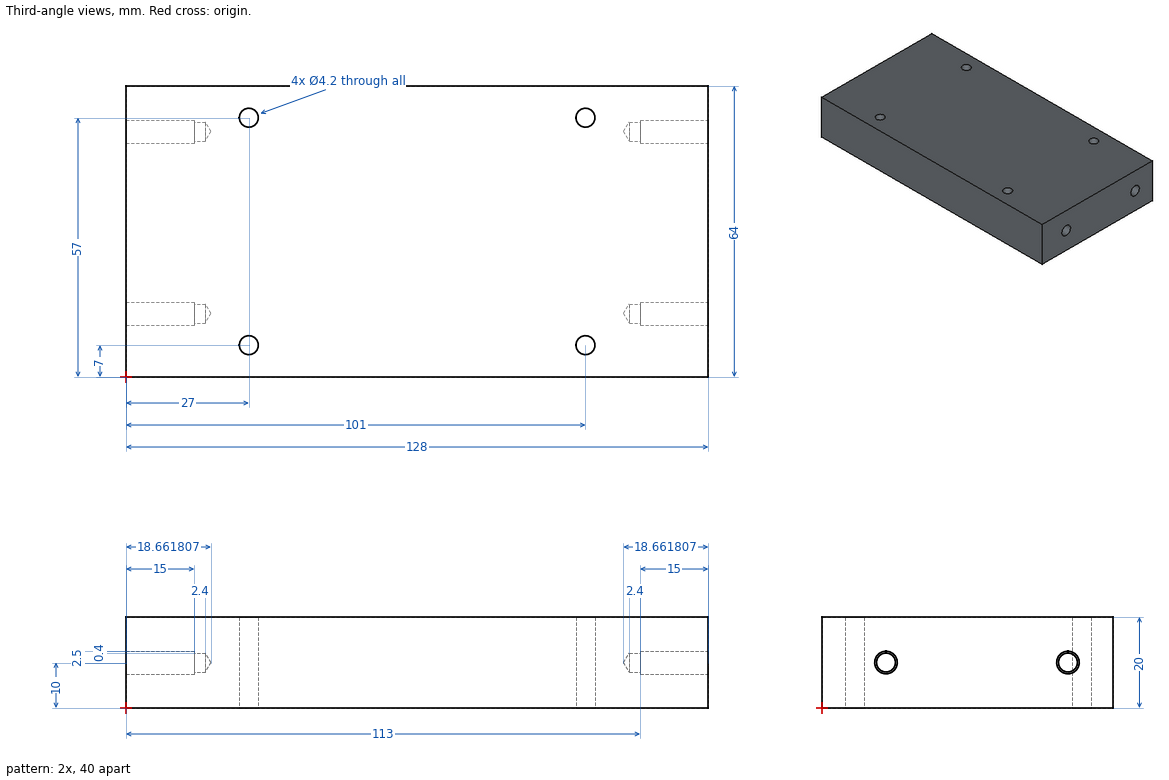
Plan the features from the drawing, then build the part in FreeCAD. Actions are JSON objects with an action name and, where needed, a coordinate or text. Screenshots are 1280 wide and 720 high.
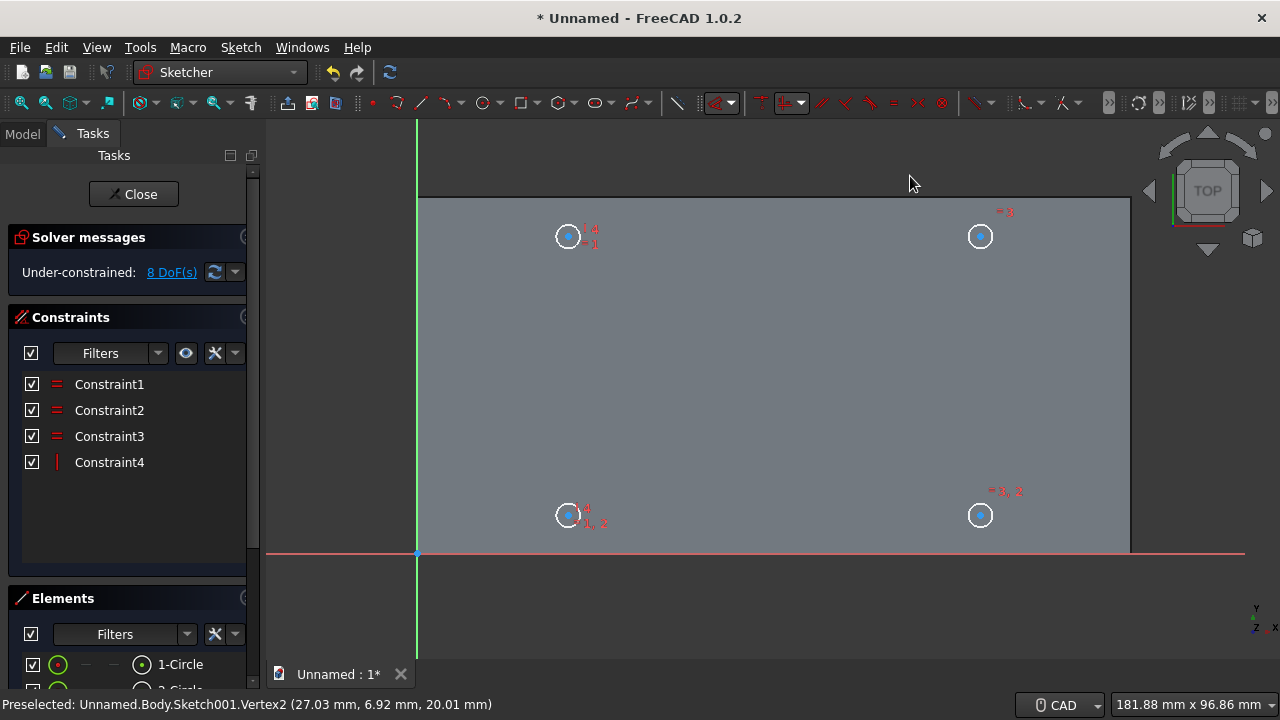
{"action": "left_click", "coordinate": [568, 515]}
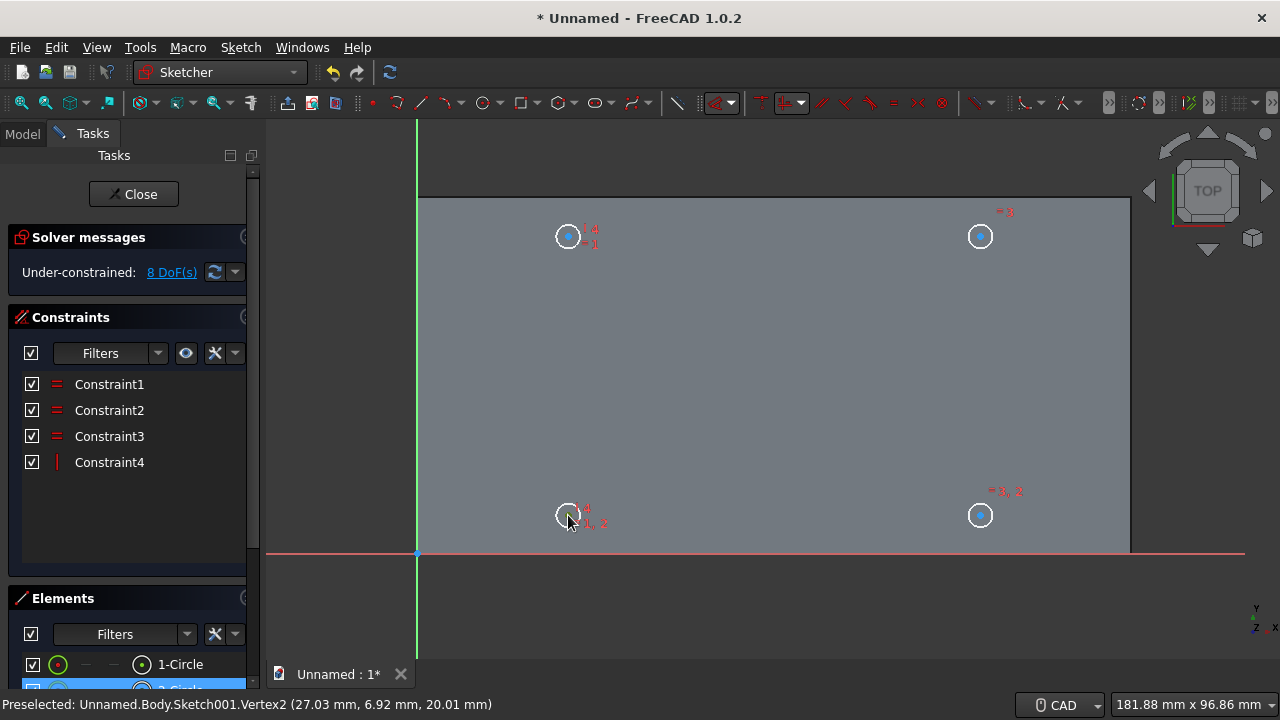
{"action": "left_click", "coordinate": [980, 515]}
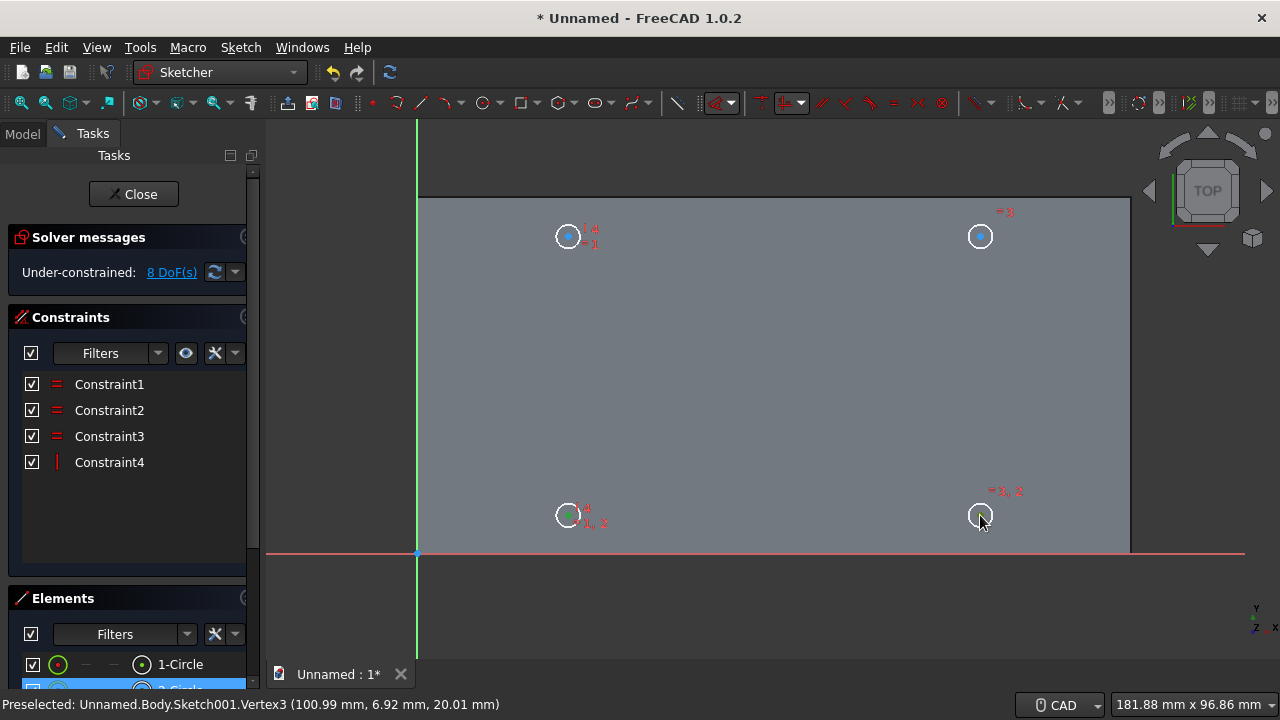
{"action": "left_click", "coordinate": [804, 104]}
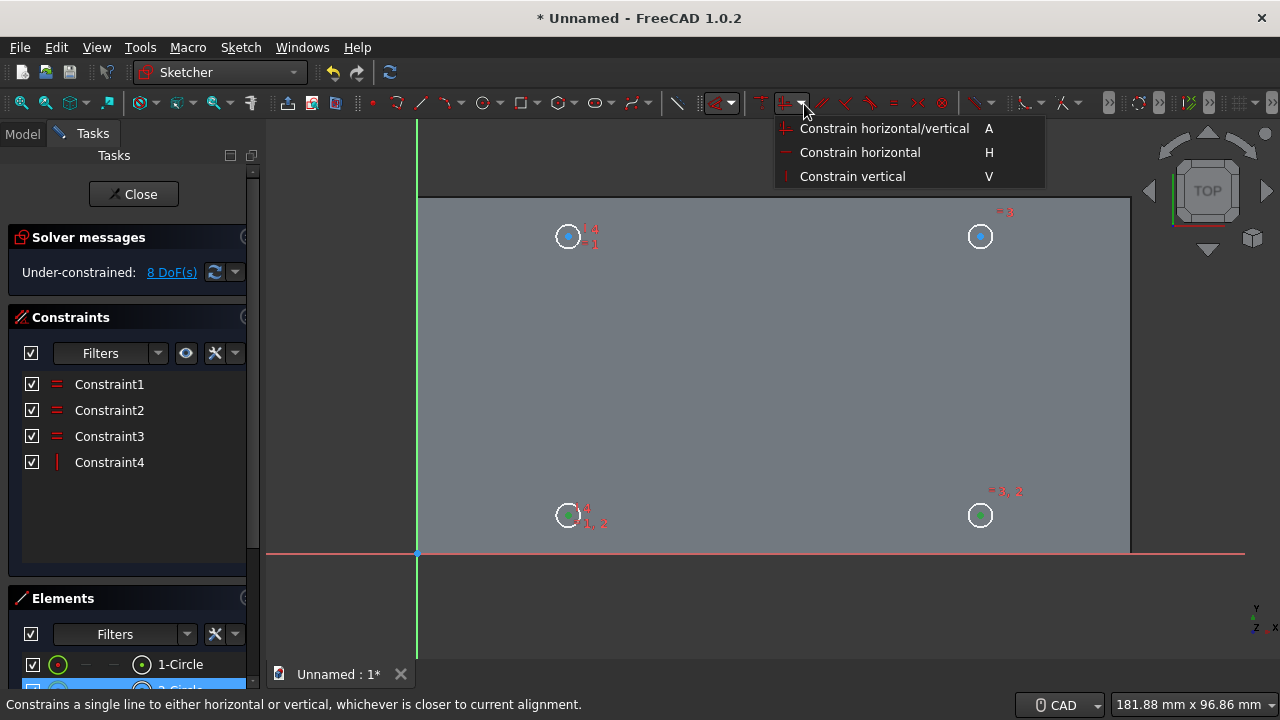
{"action": "left_click", "coordinate": [910, 152]}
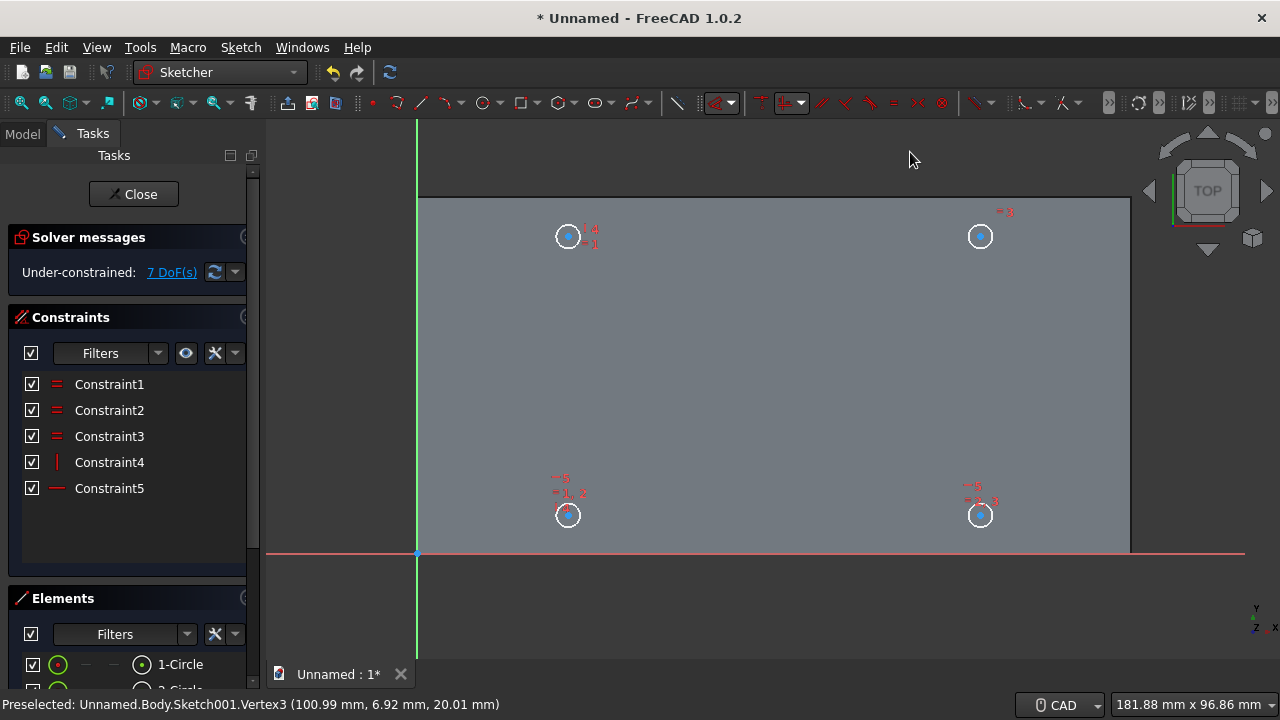
{"action": "left_click", "coordinate": [980, 515]}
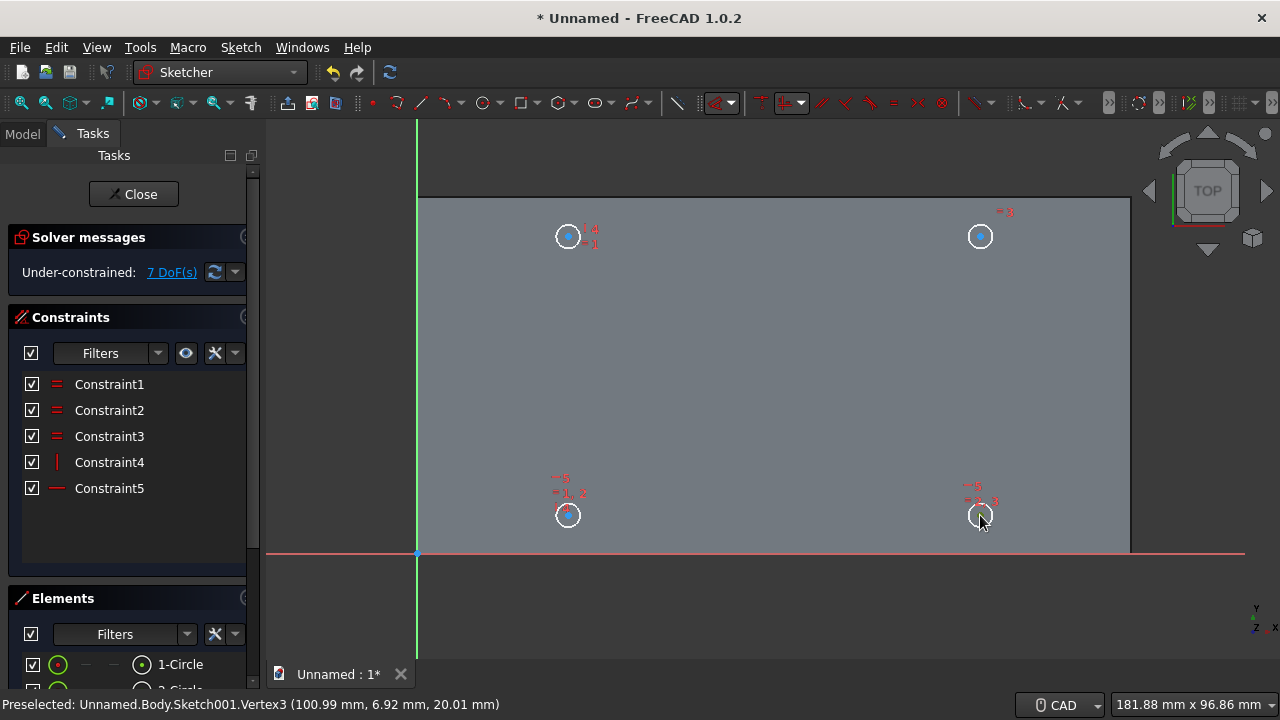
{"action": "left_click", "coordinate": [980, 237]}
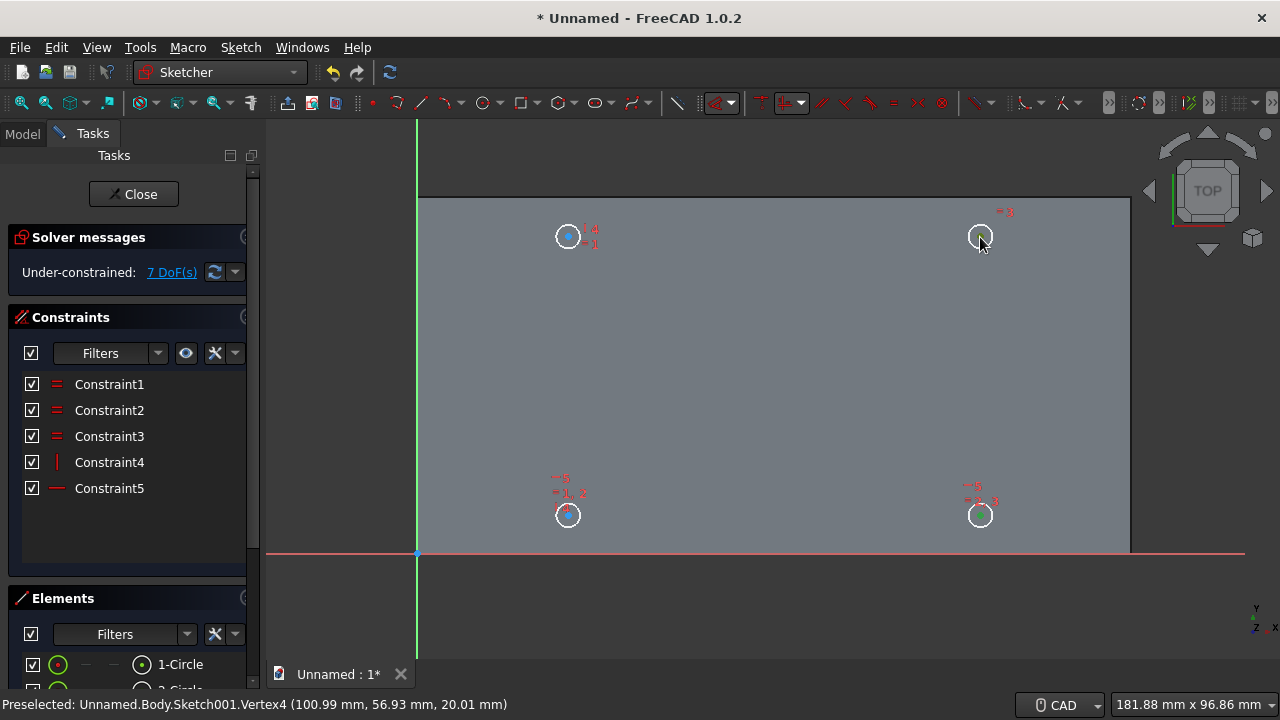
{"action": "key", "text": "v"}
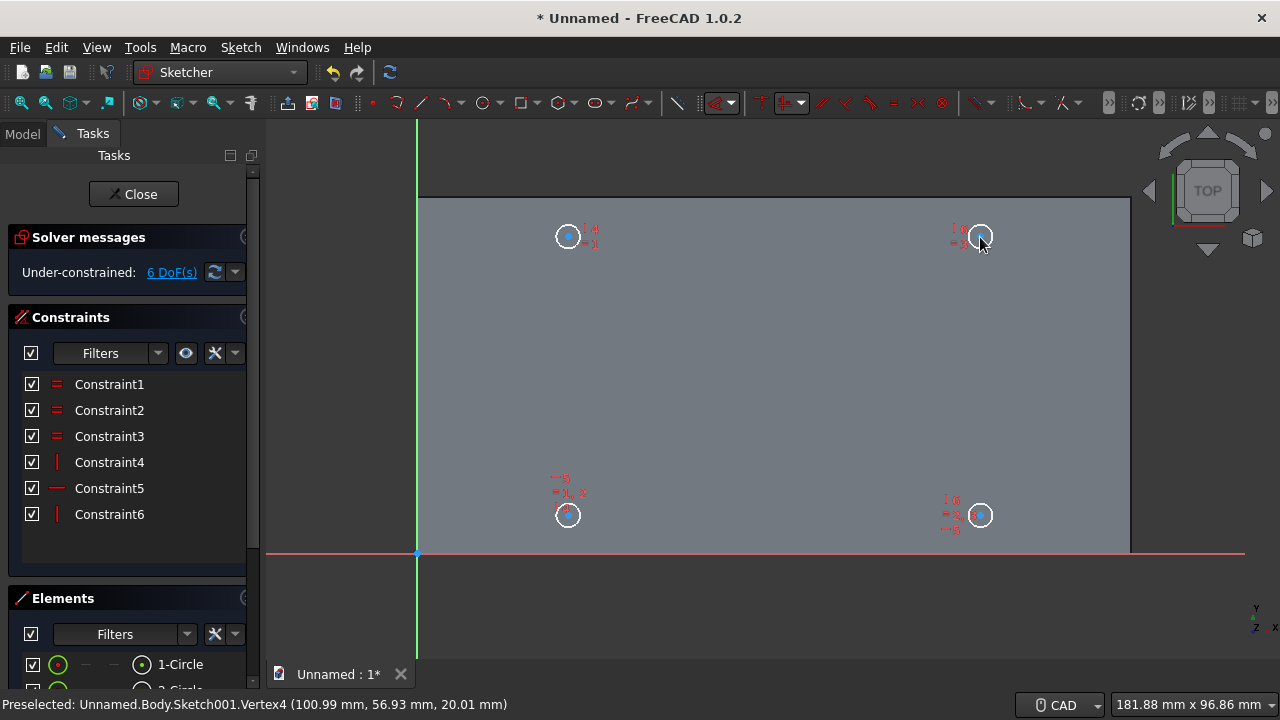
{"action": "left_click", "coordinate": [568, 237]}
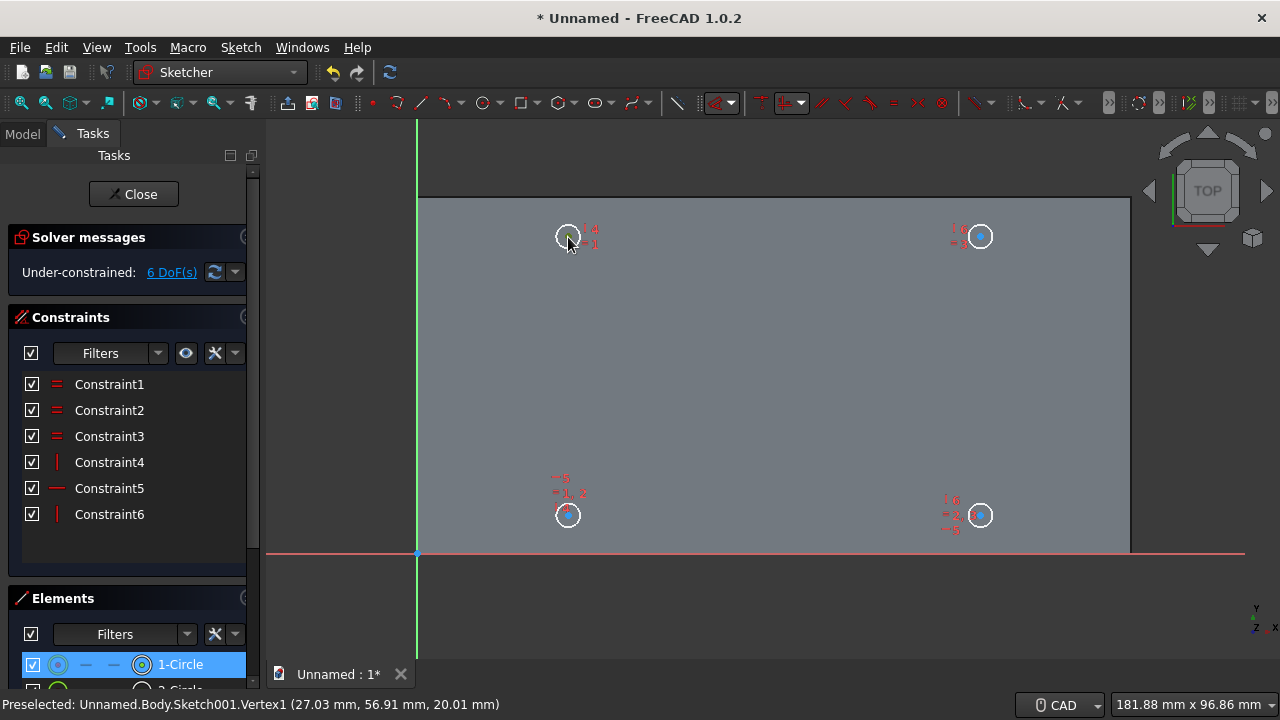
{"action": "left_click", "coordinate": [980, 237]}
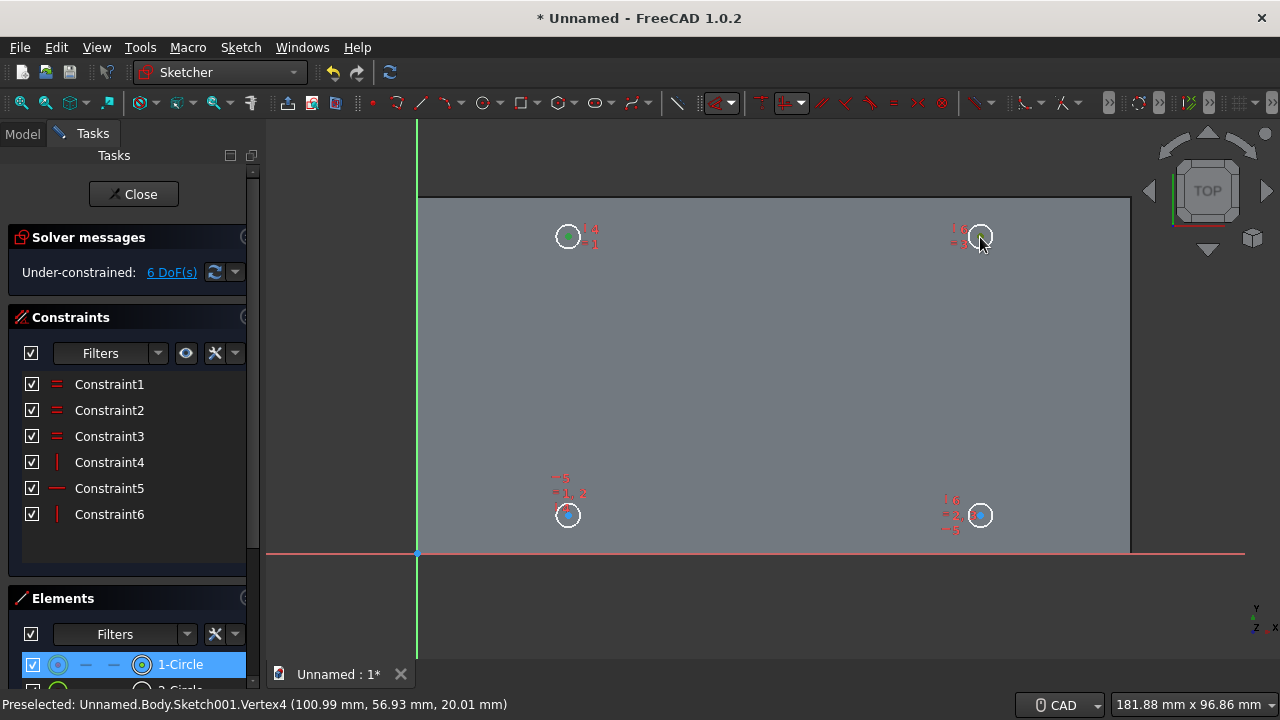
{"action": "left_click", "coordinate": [804, 104]}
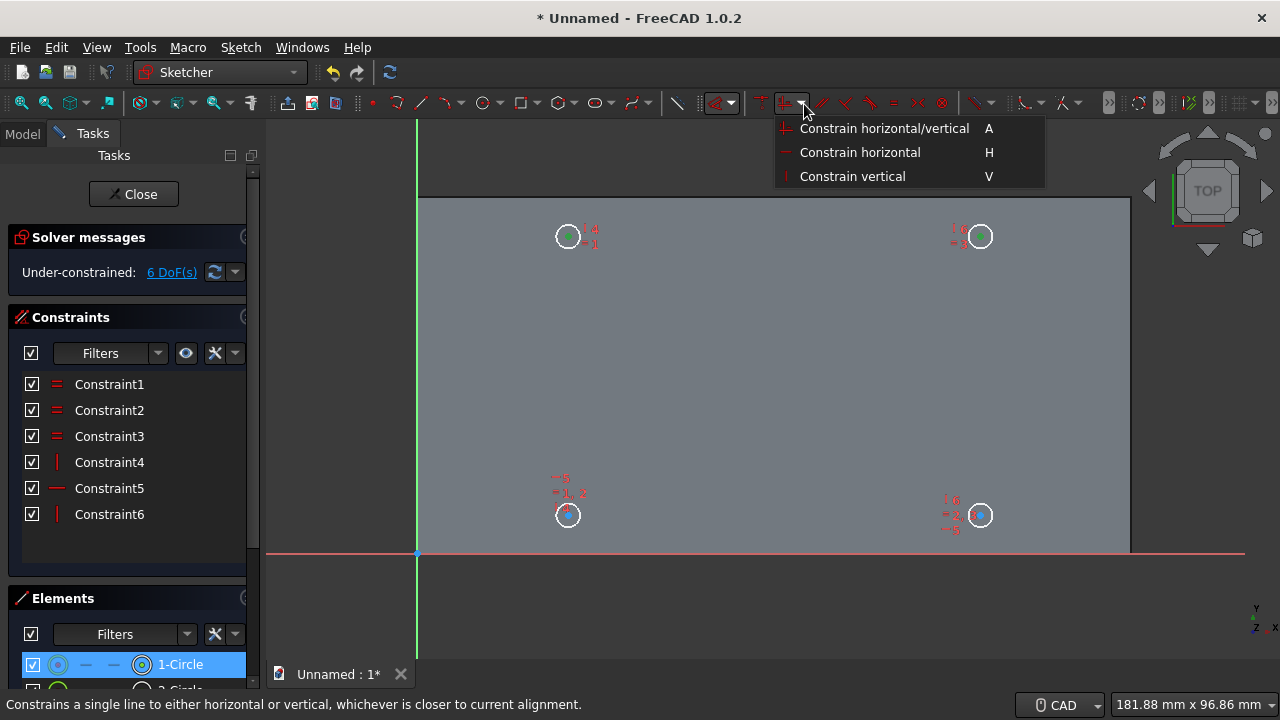
{"action": "left_click", "coordinate": [910, 152]}